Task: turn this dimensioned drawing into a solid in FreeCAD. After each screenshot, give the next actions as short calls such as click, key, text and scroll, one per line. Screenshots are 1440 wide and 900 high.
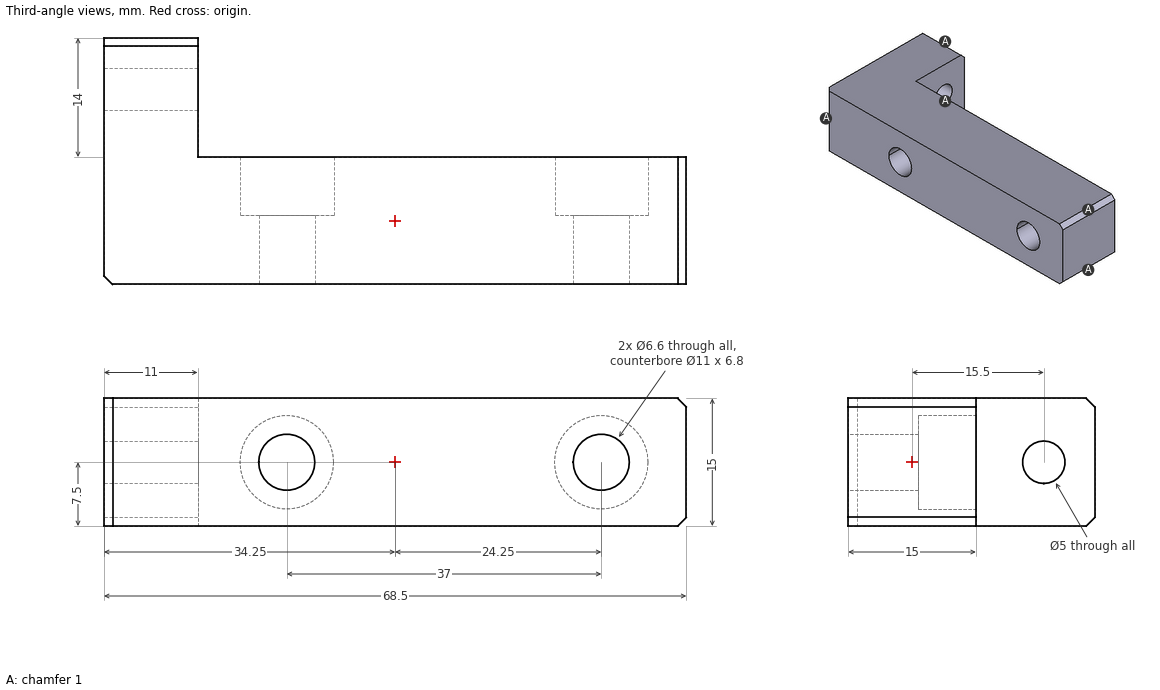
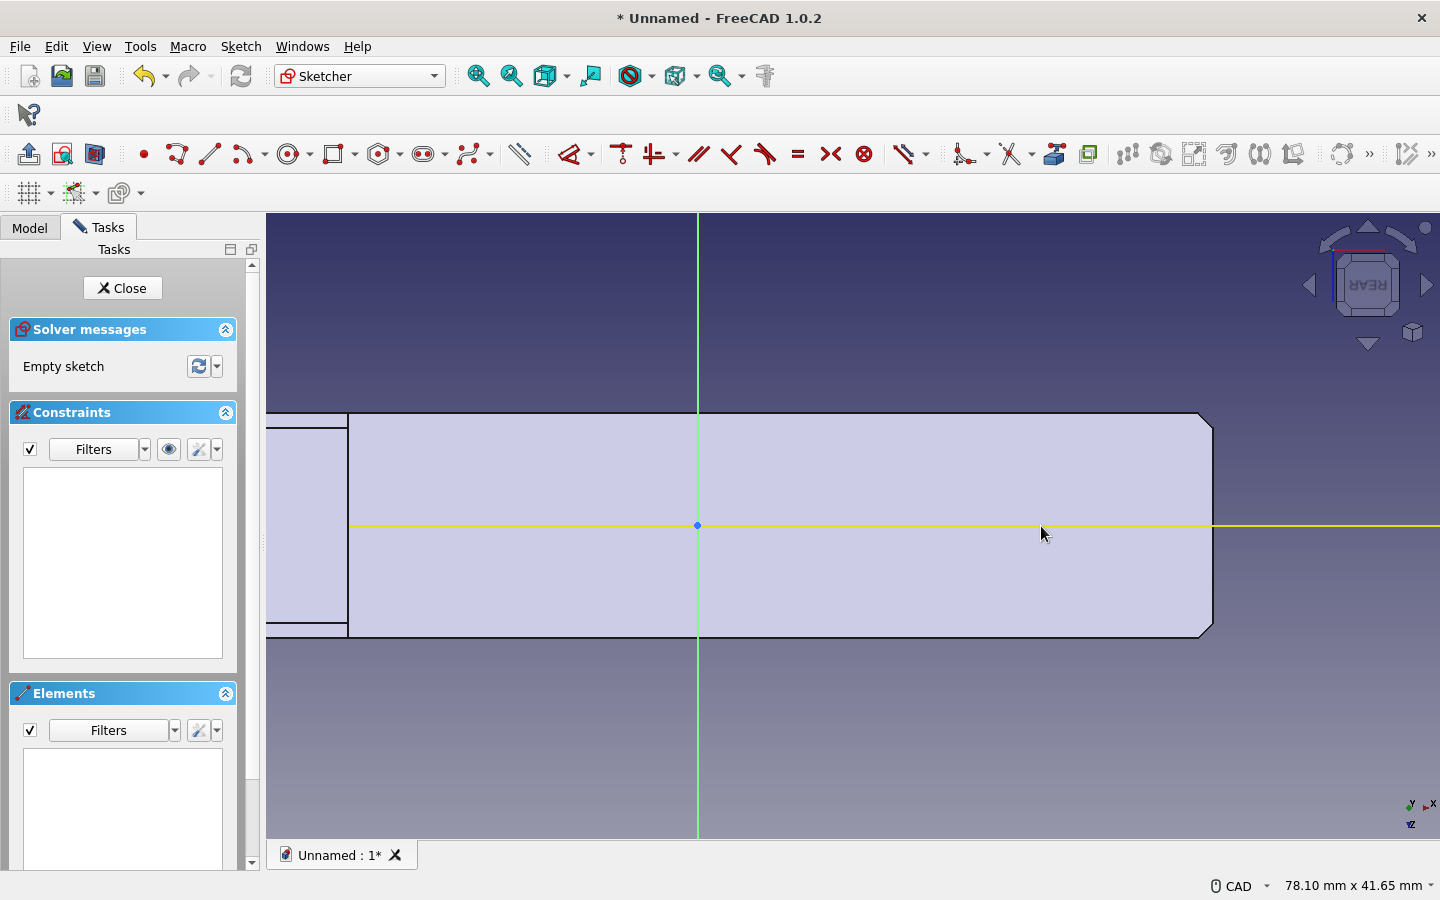
click(288, 154)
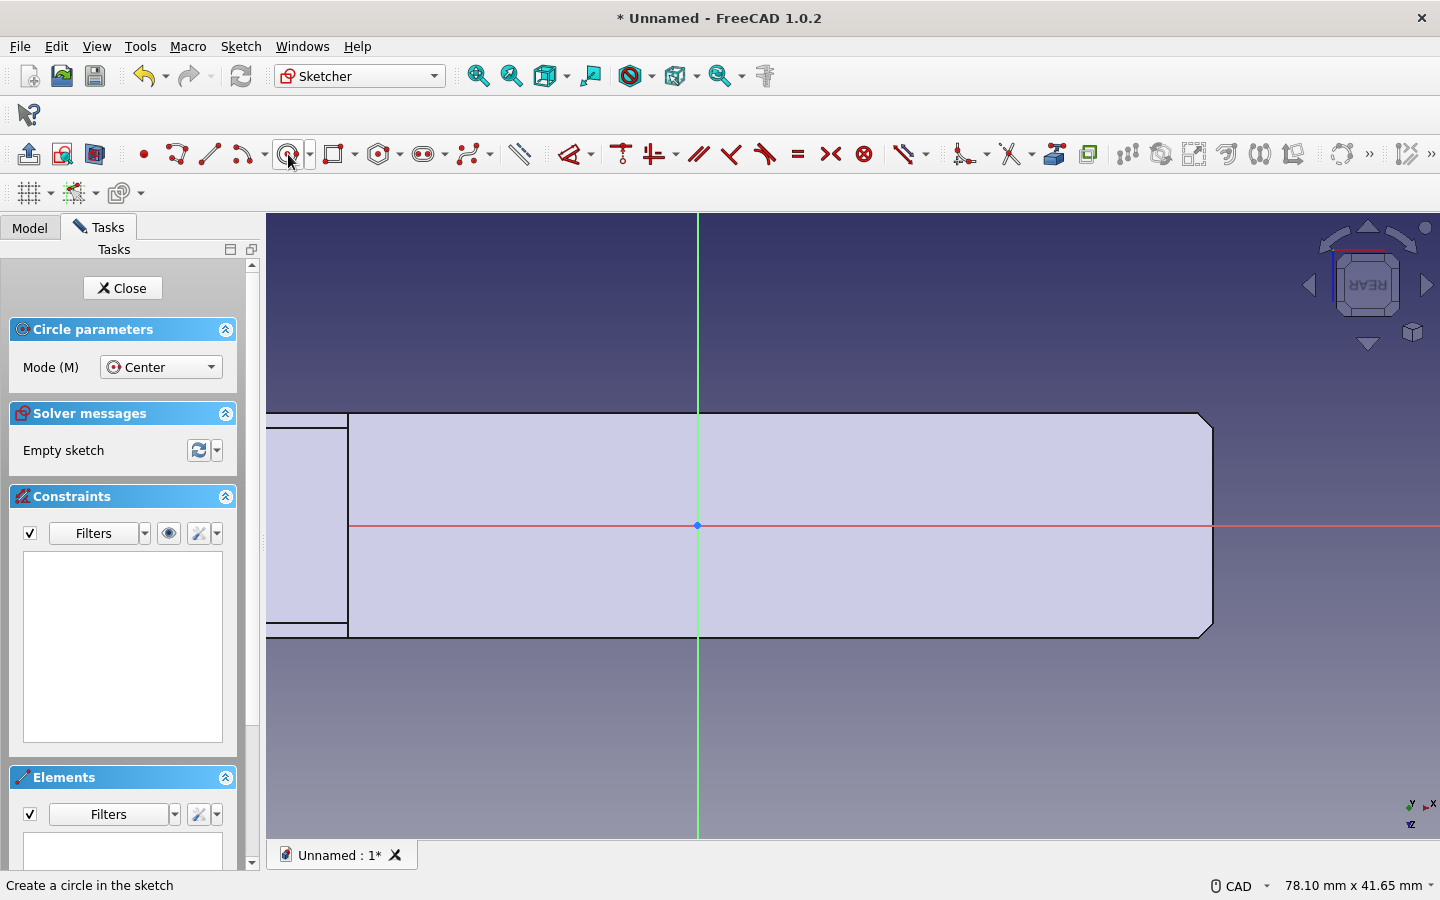
click(1062, 526)
move(1097, 491)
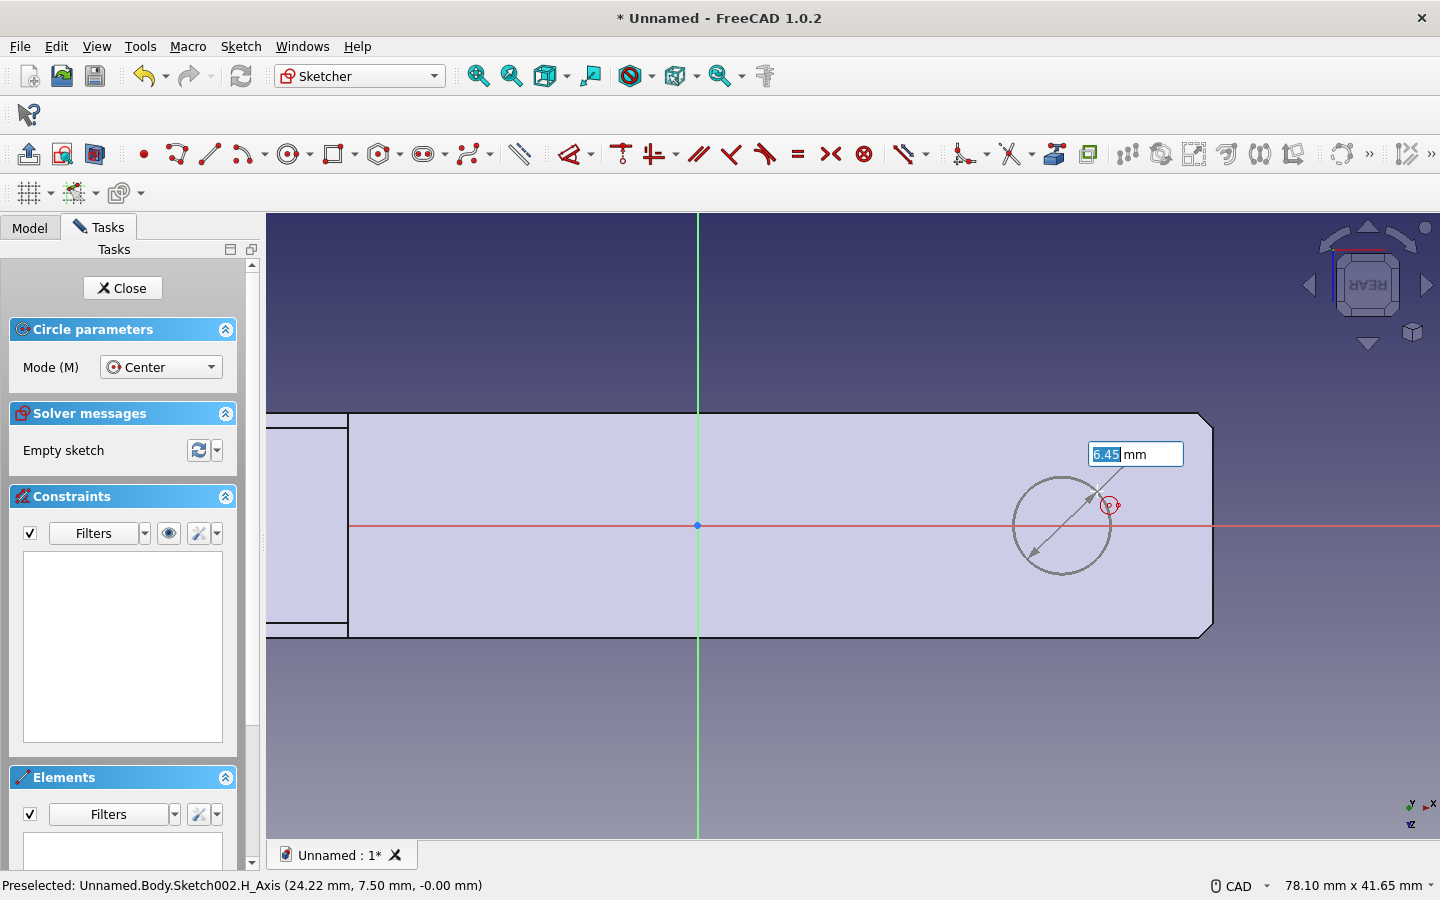
text(6.6)
key(Return)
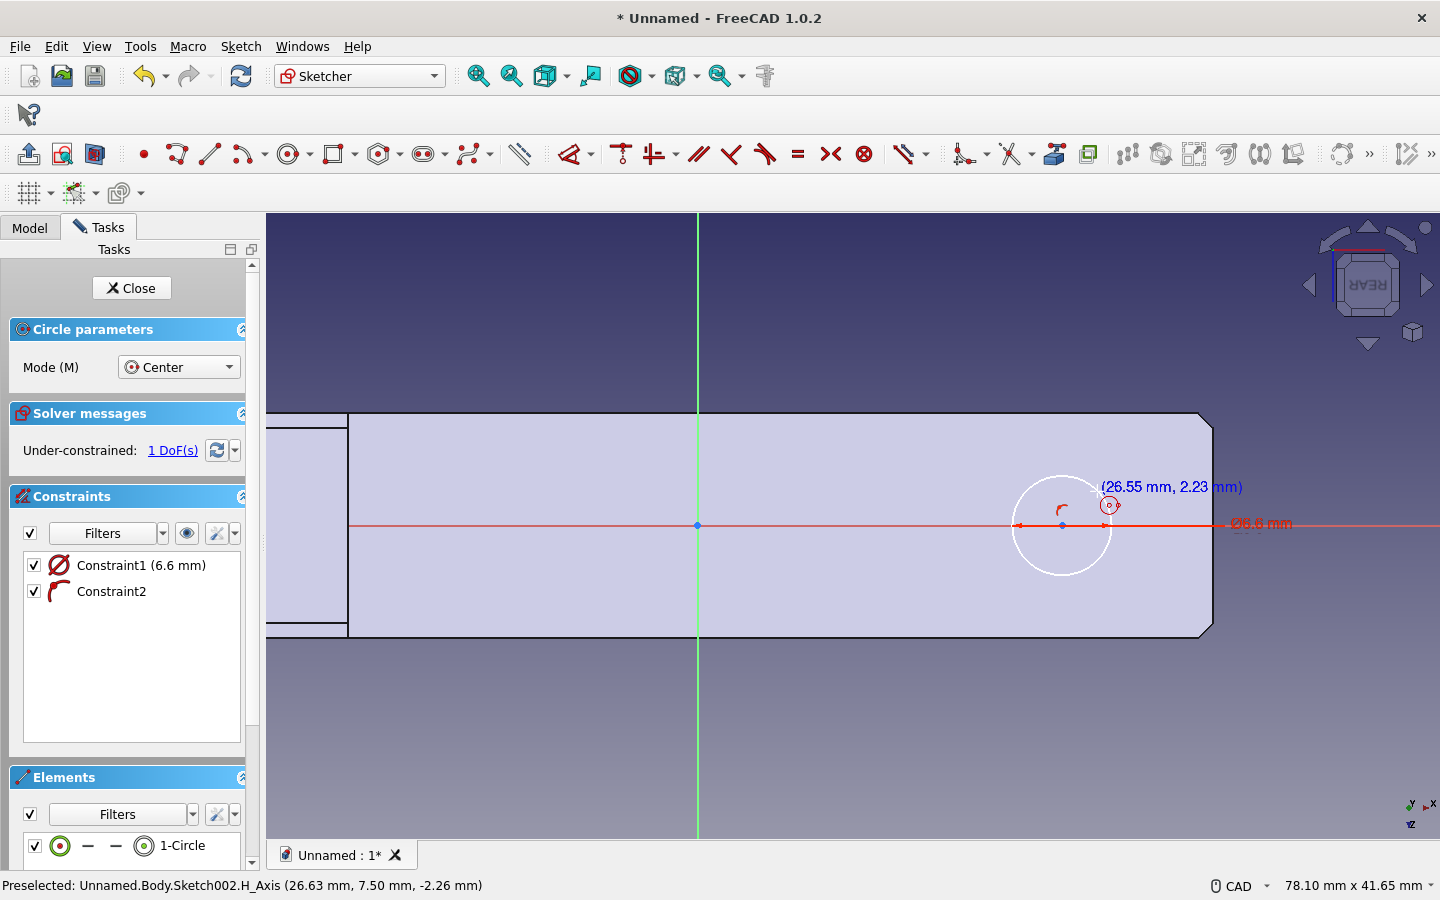
click(506, 526)
move(541, 491)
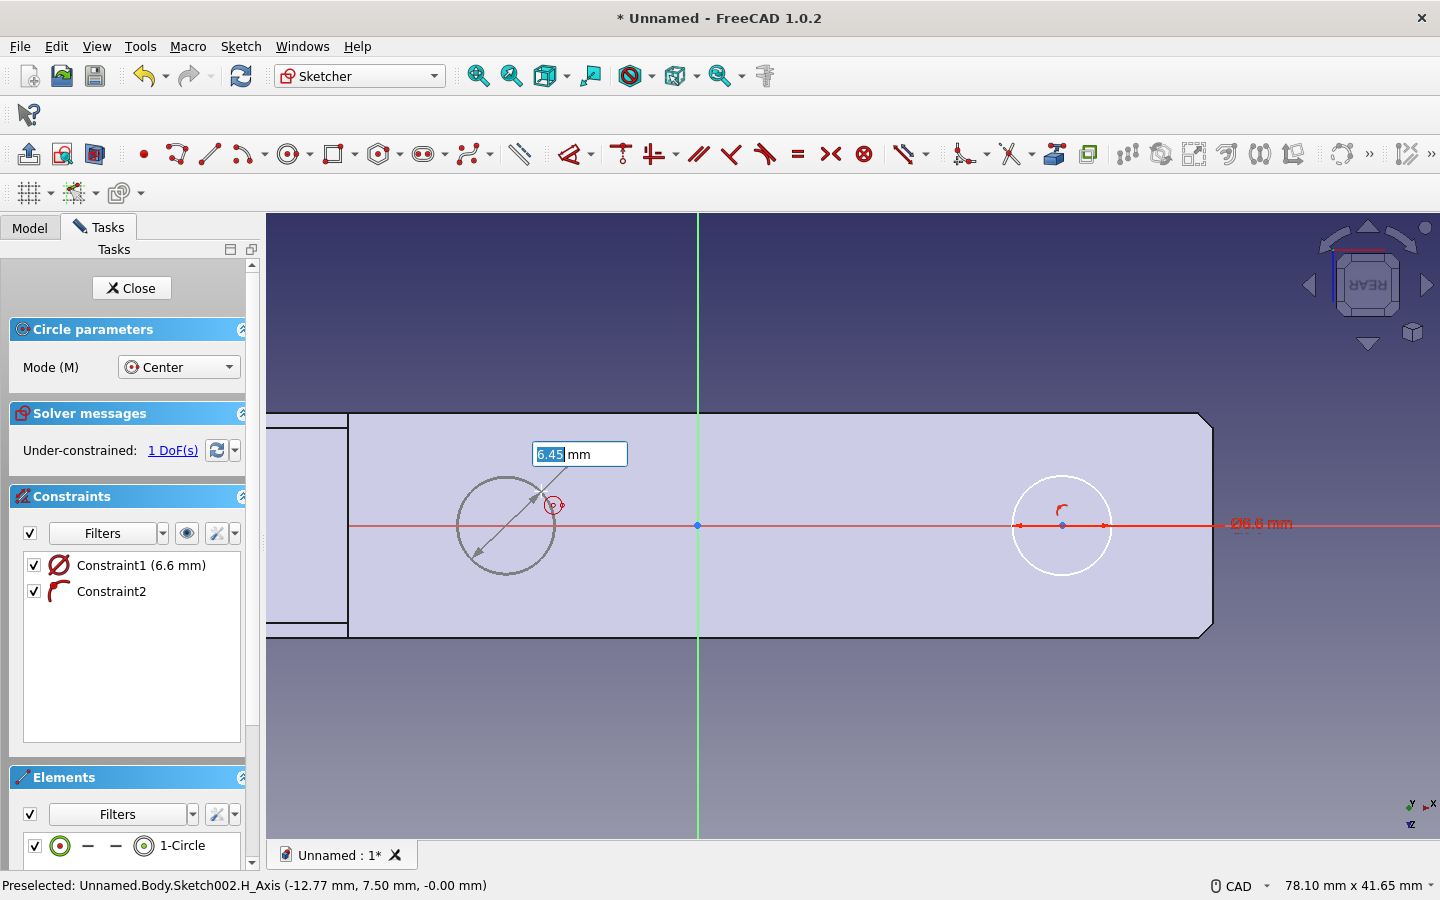
text(6.6)
key(Return)
key(Escape)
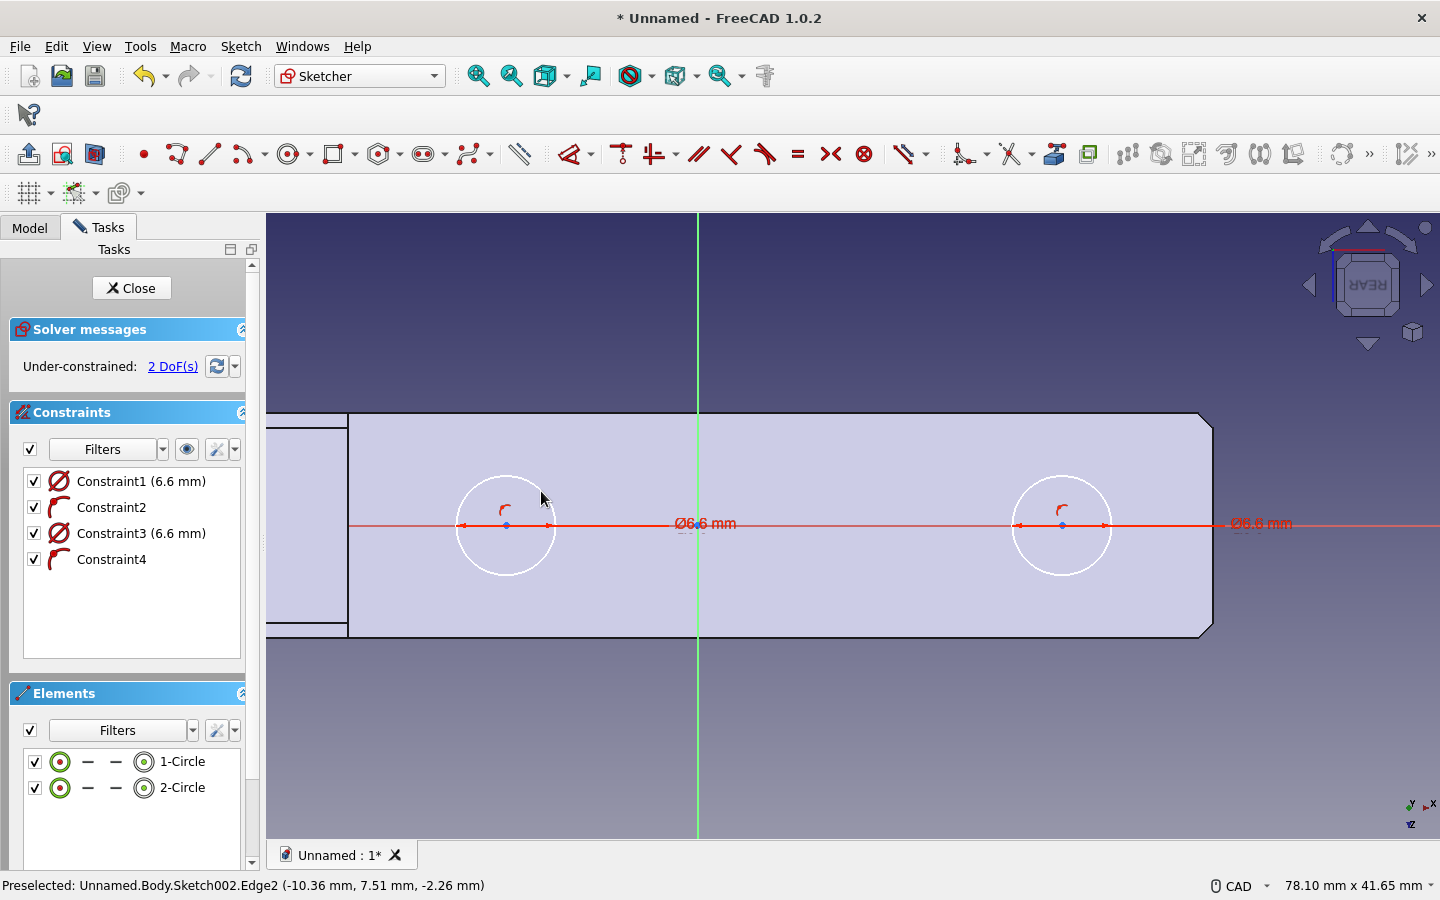
click(568, 154)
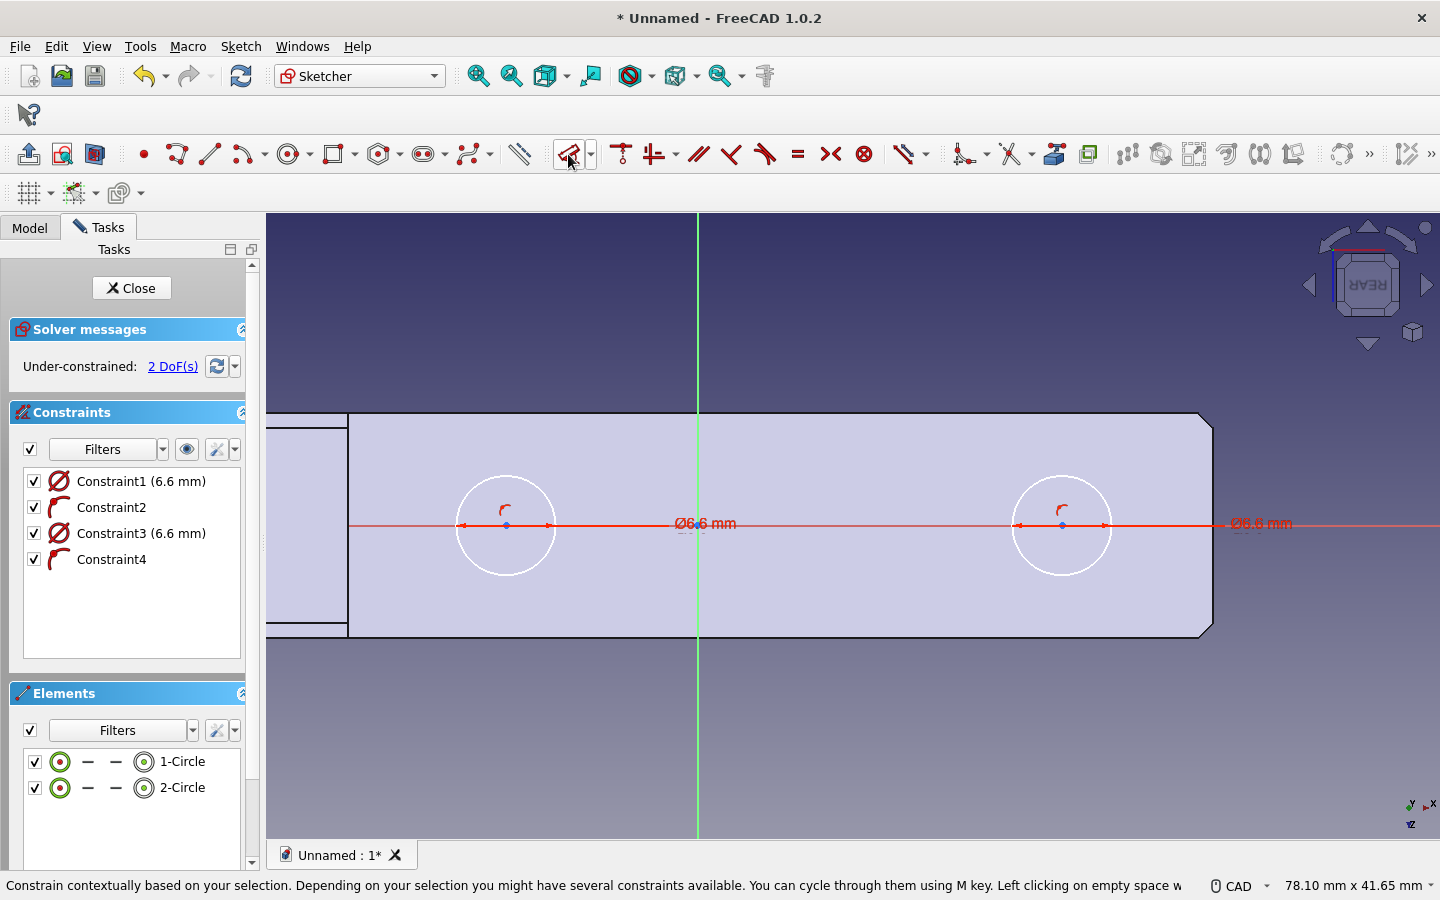
click(1062, 526)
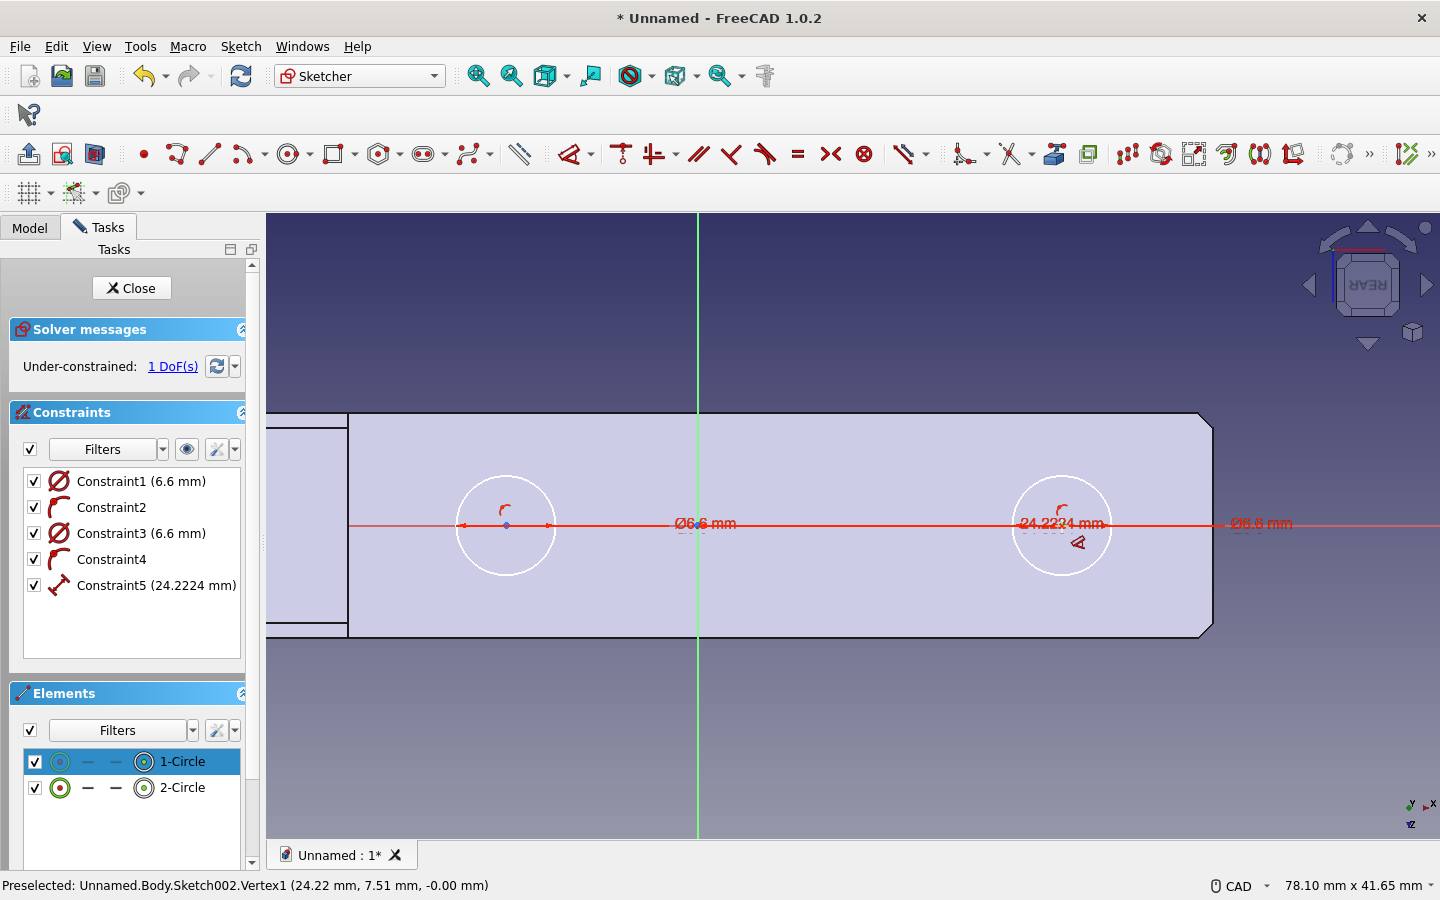
click(506, 526)
click(784, 560)